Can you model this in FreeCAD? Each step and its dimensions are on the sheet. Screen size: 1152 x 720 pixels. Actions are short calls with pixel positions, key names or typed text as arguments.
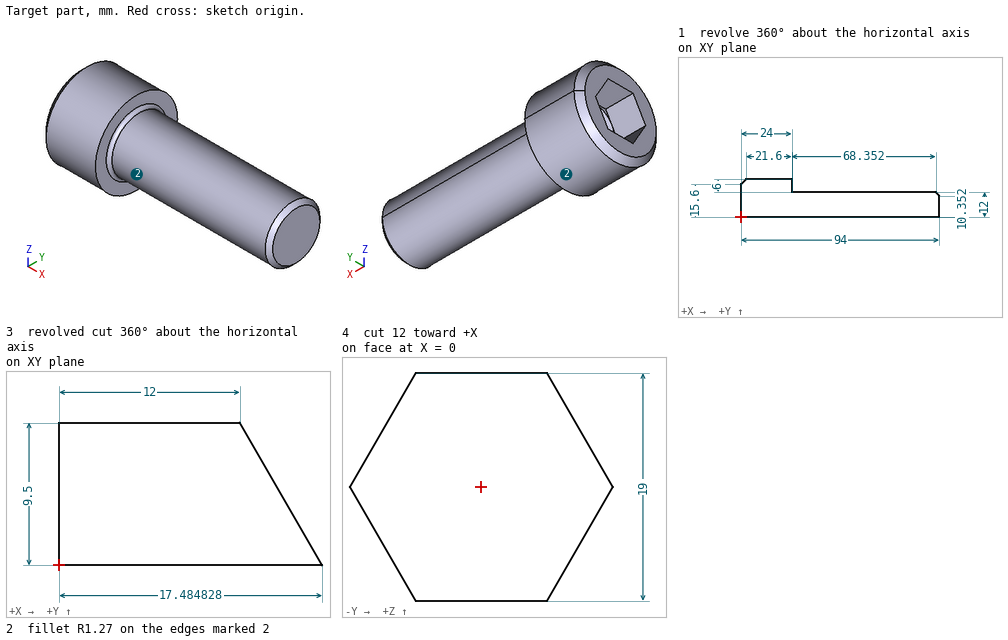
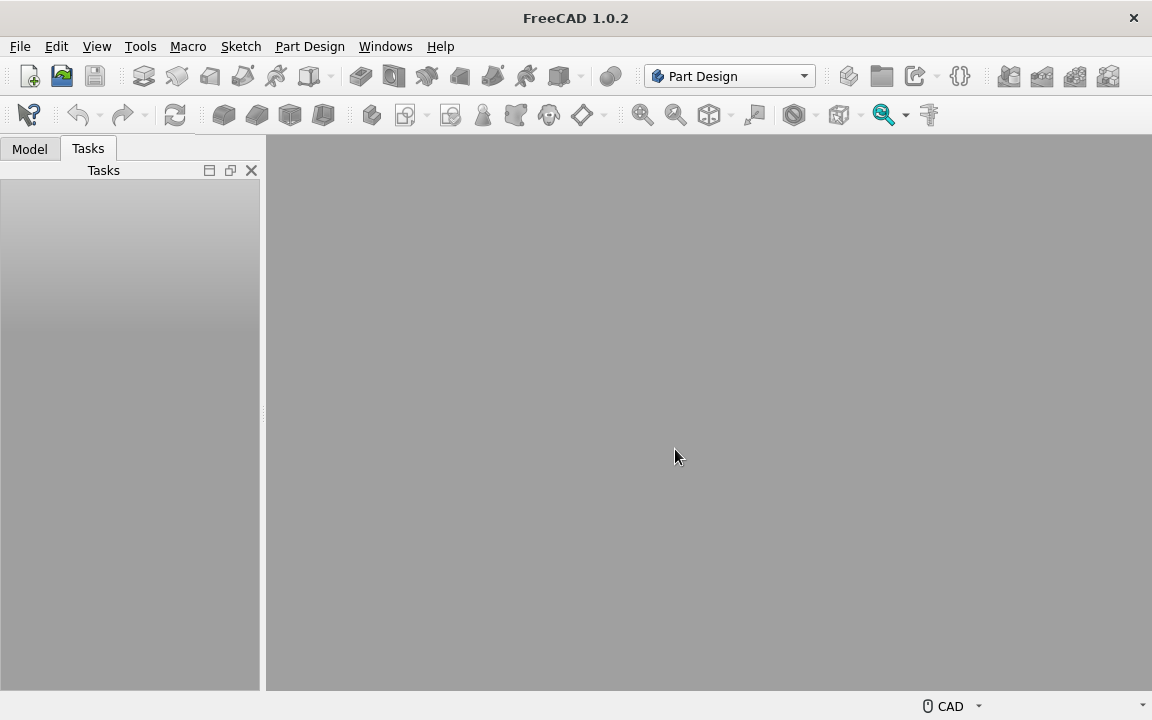
click(29, 76)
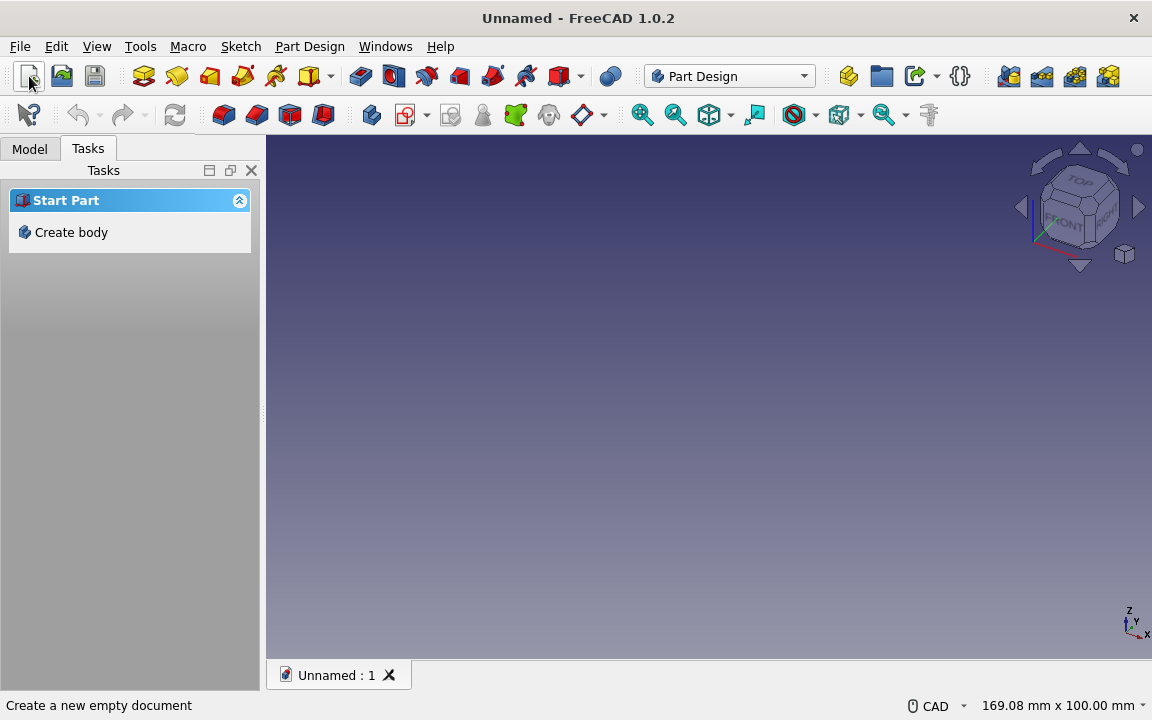
click(404, 116)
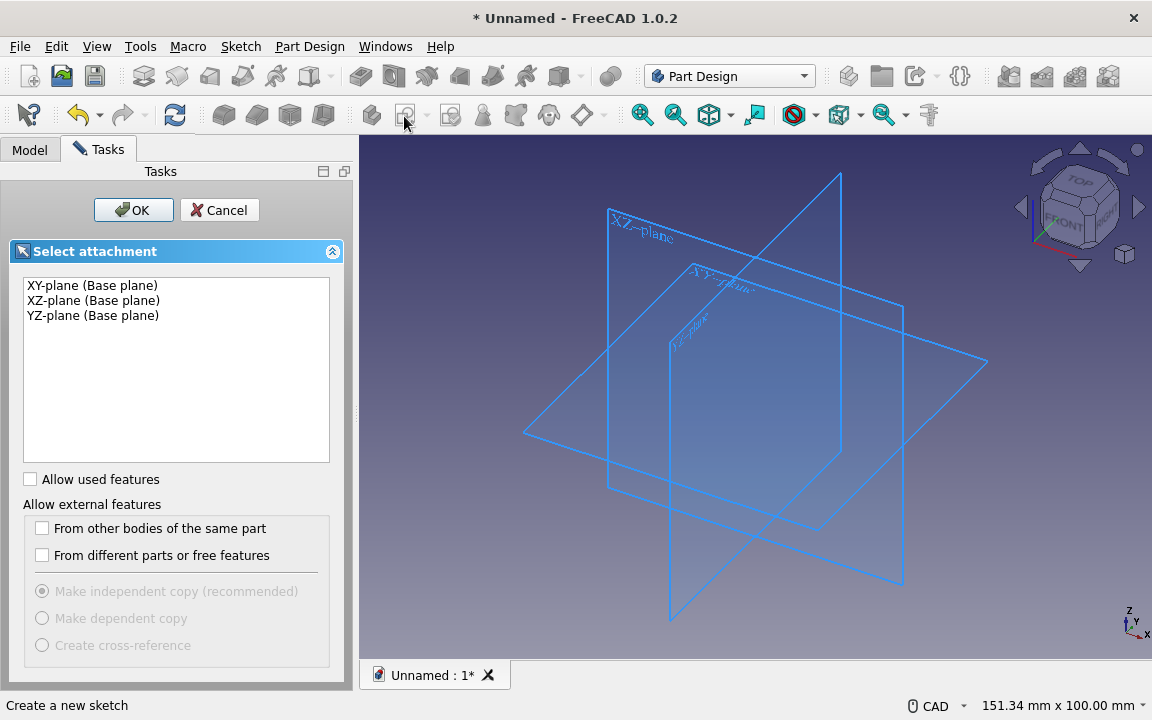
click(84, 286)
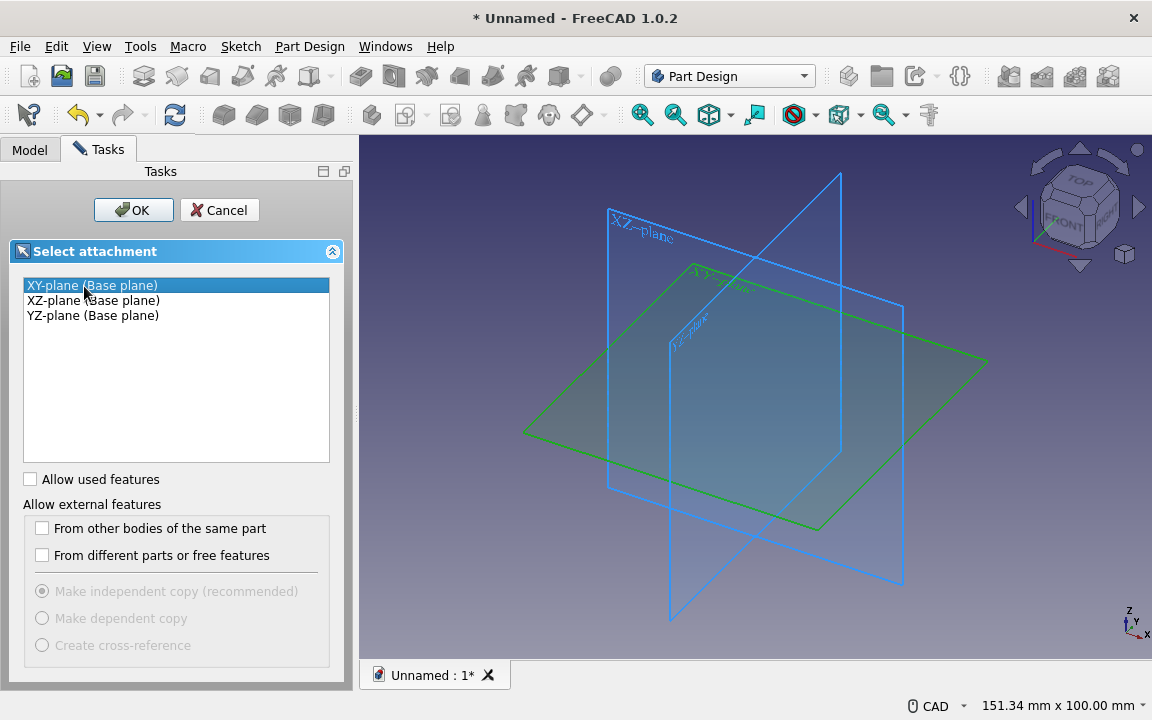
click(134, 210)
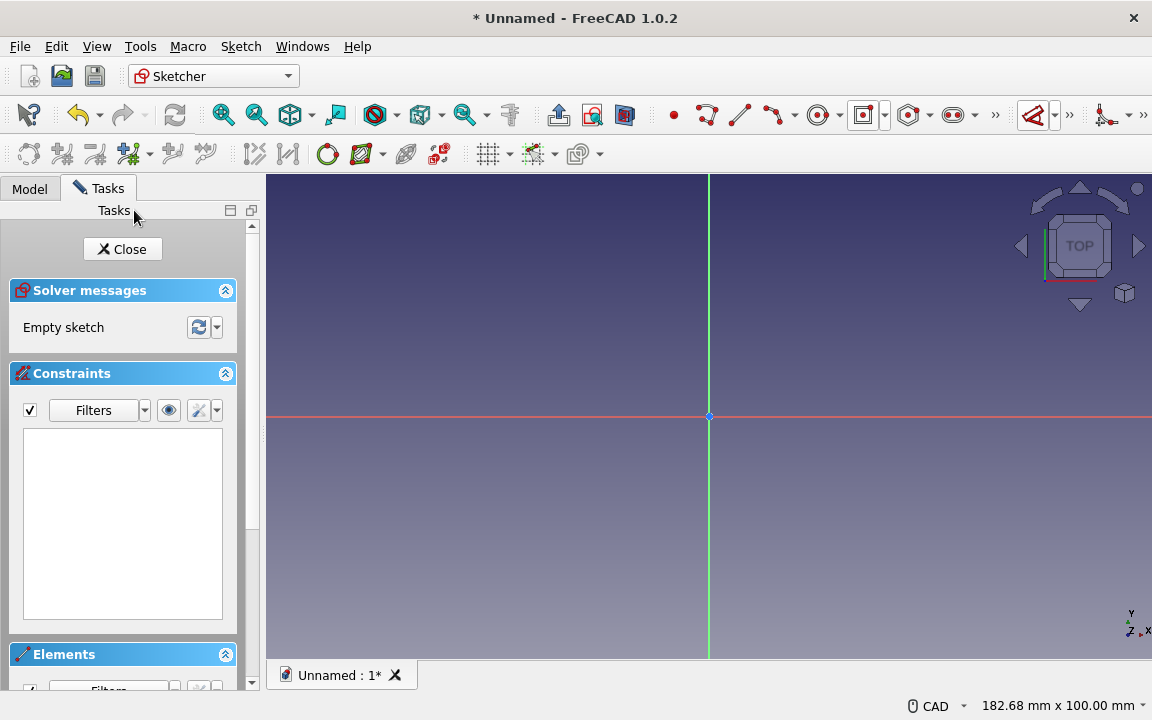
scroll(294, 505, down, 2)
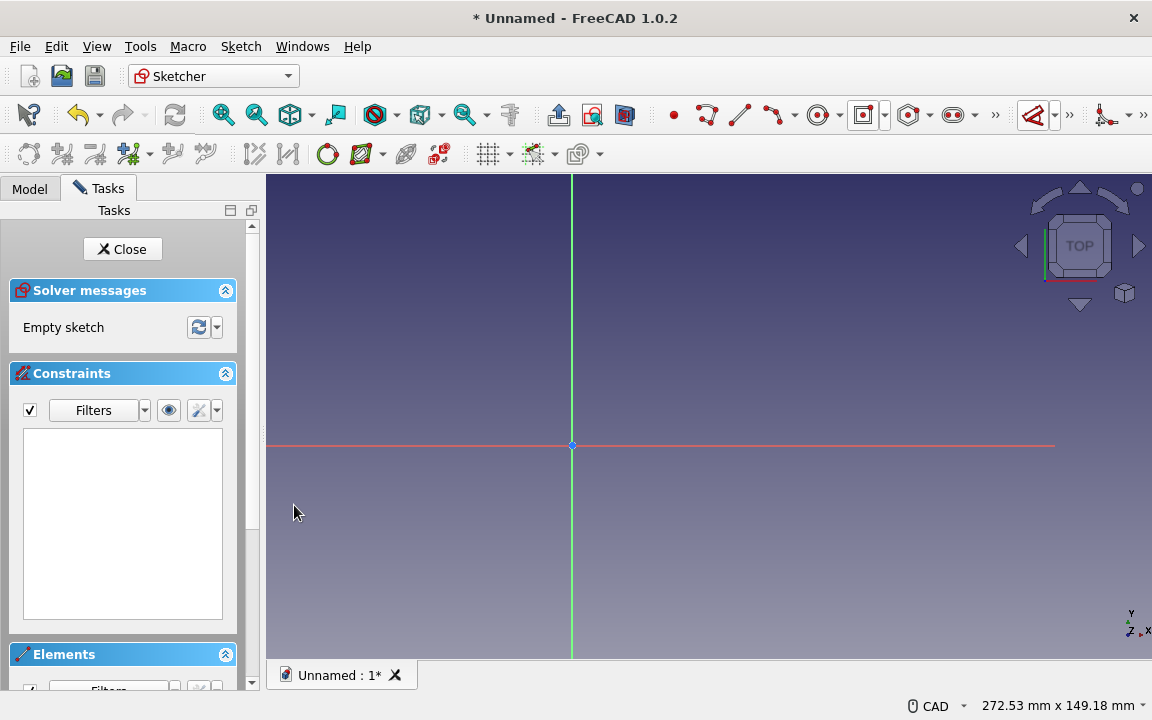
scroll(897, 417, up, 2)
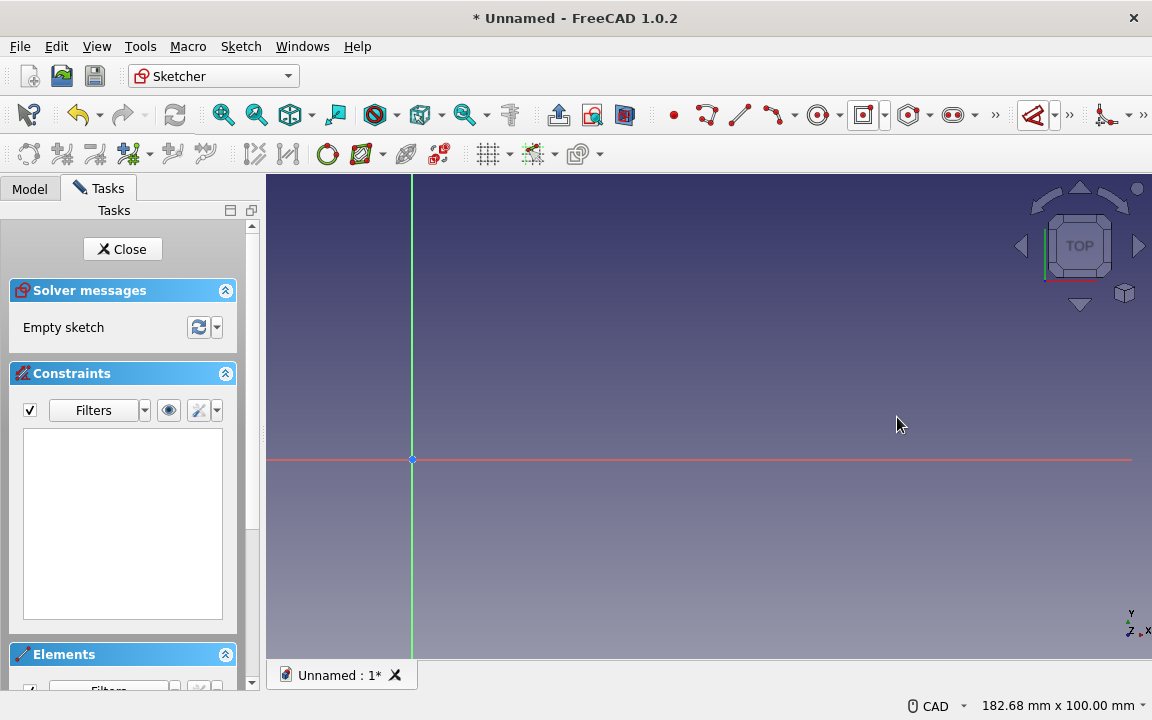
click(707, 116)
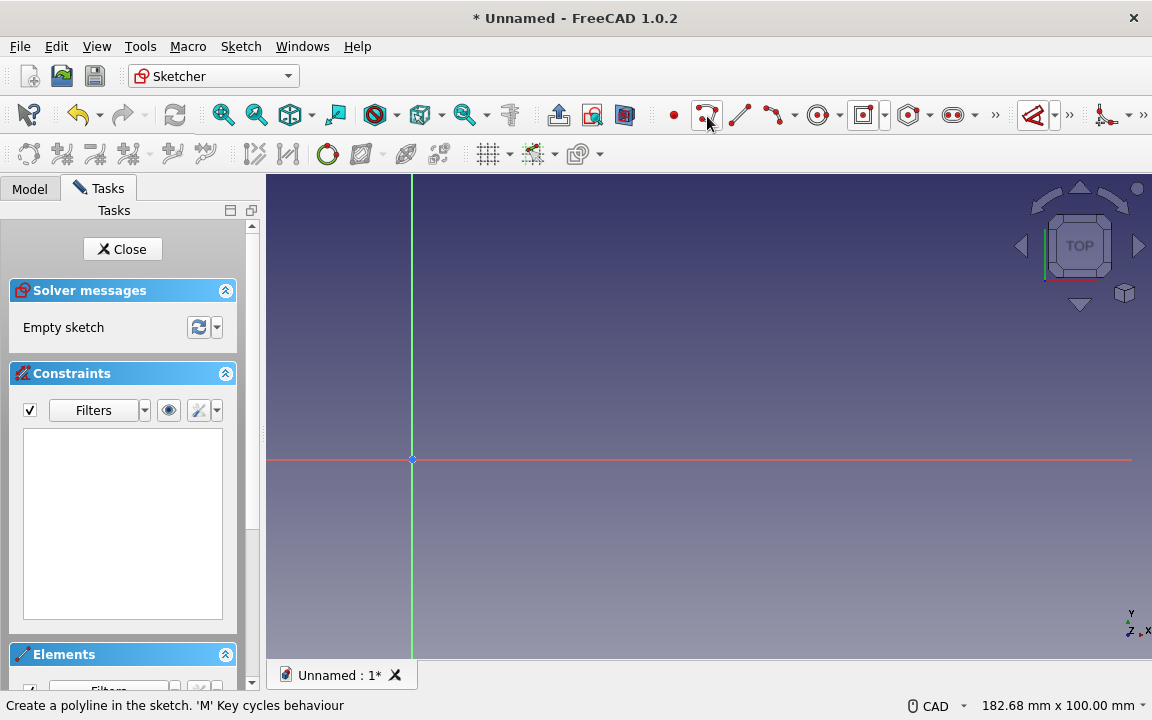
click(412, 460)
click(868, 451)
click(868, 410)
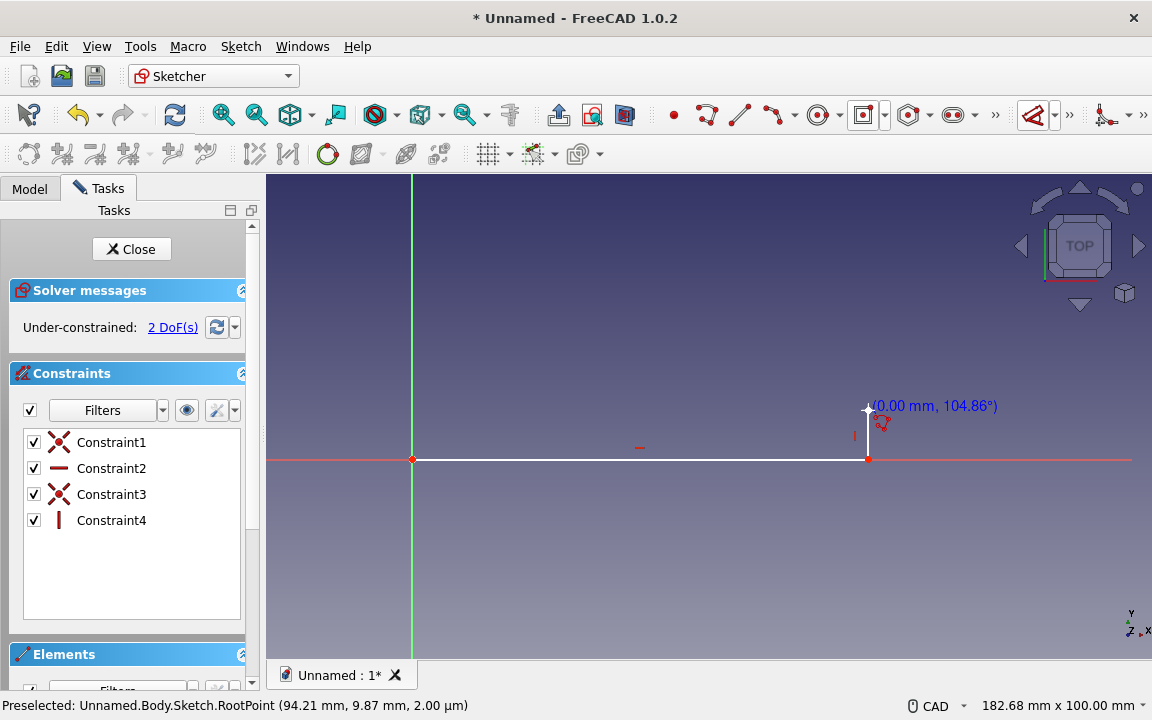
scroll(860, 402, up, 2)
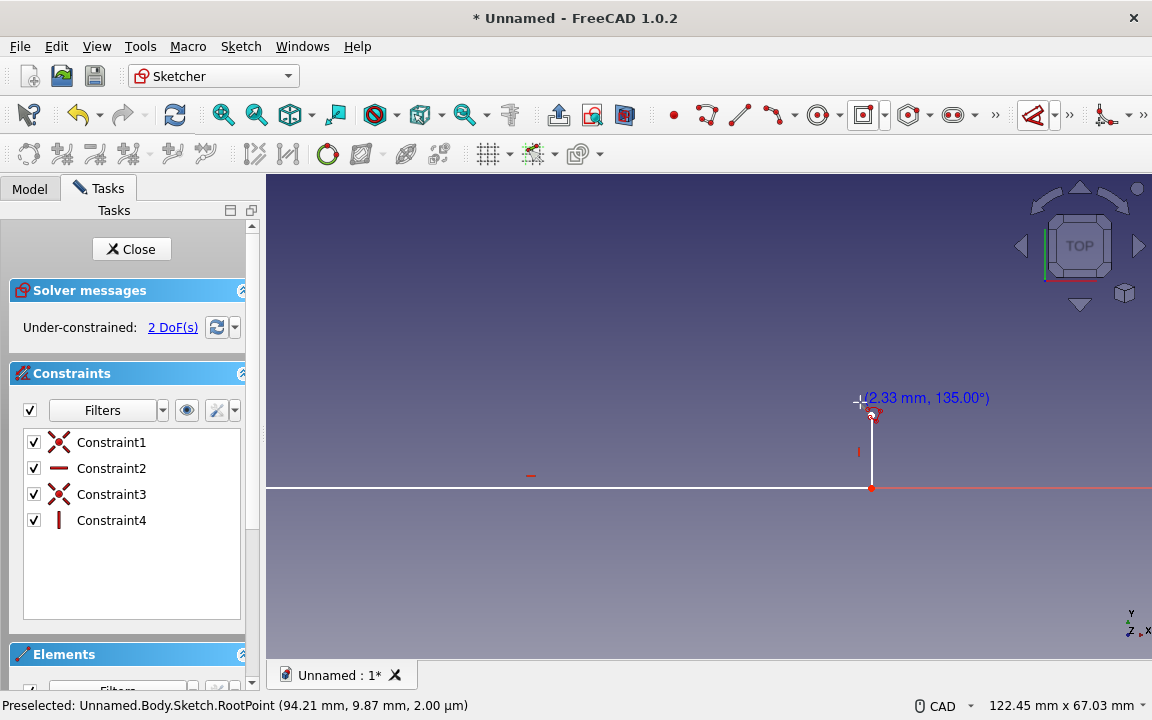
click(860, 401)
click(365, 401)
click(365, 358)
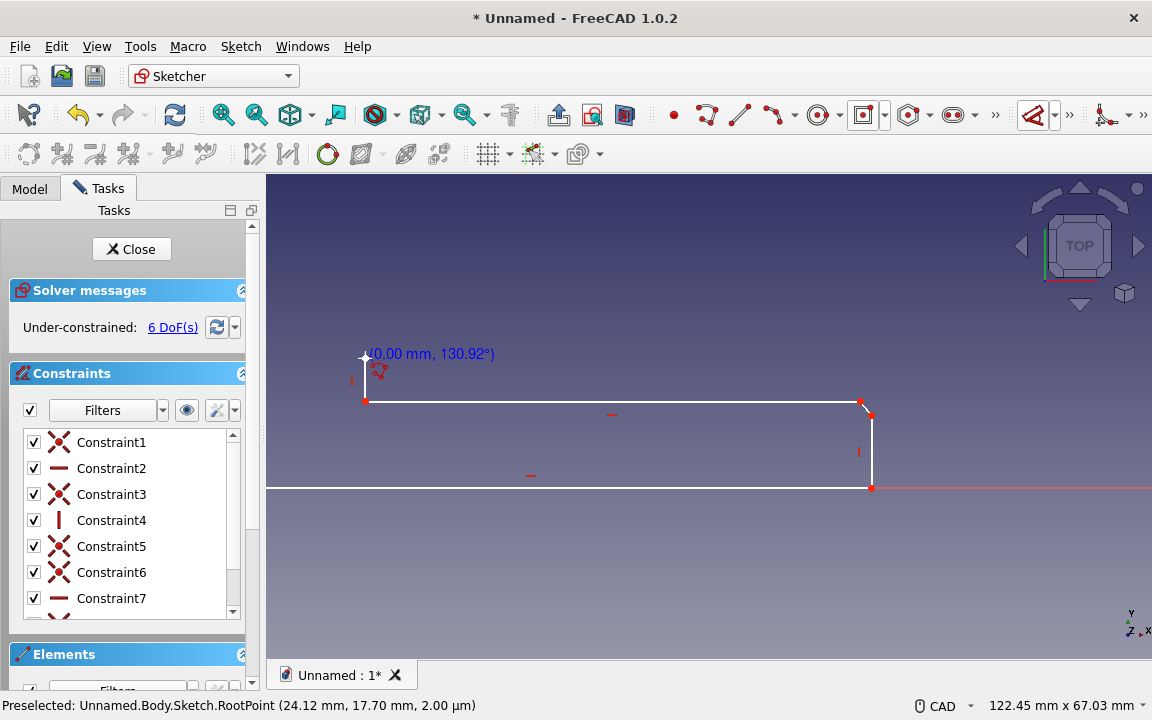
scroll(862, 403, down, 2)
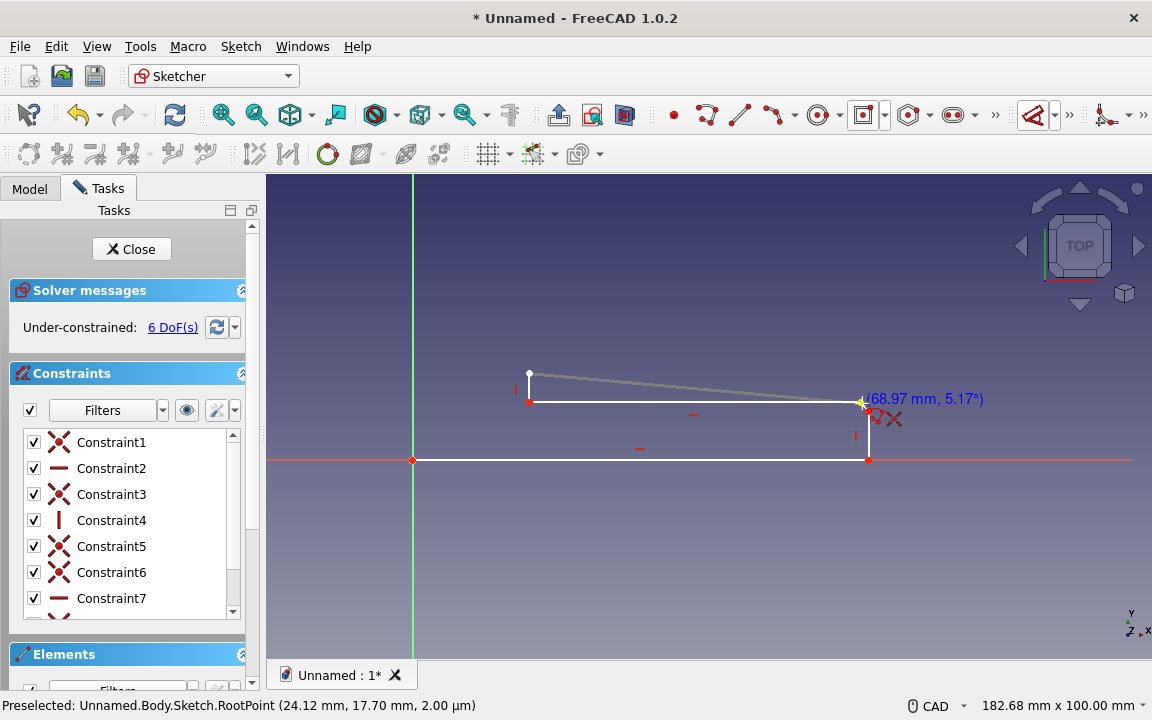
scroll(424, 373, up, 2)